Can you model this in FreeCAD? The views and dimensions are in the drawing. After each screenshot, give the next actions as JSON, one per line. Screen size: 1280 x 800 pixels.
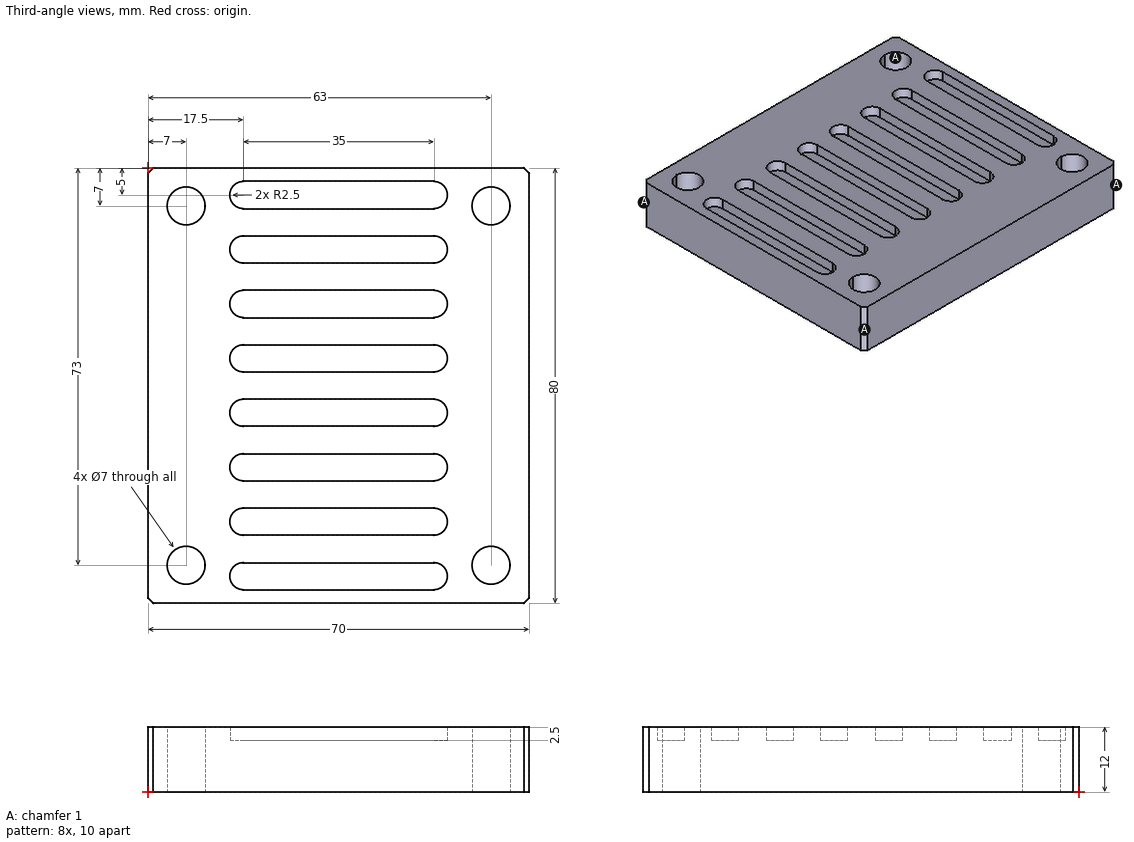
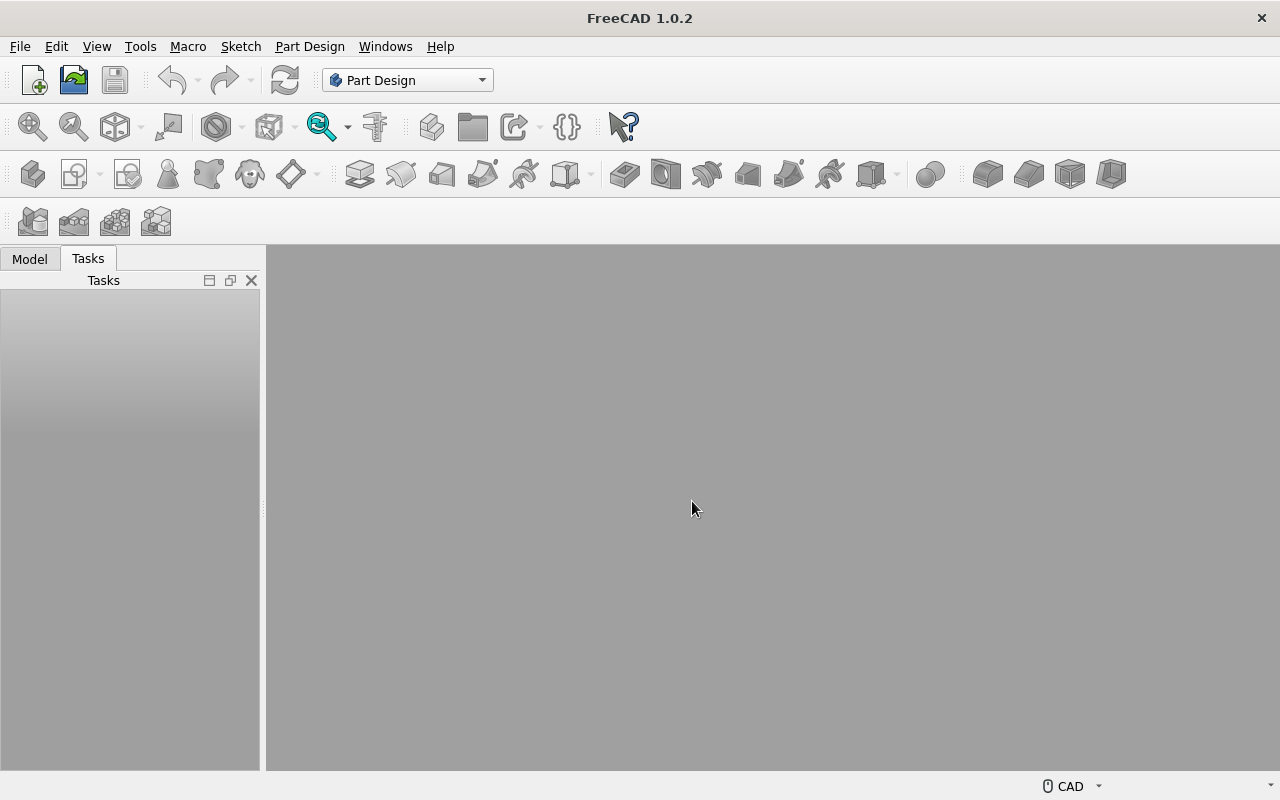
{"action": "key", "text": "ctrl+n"}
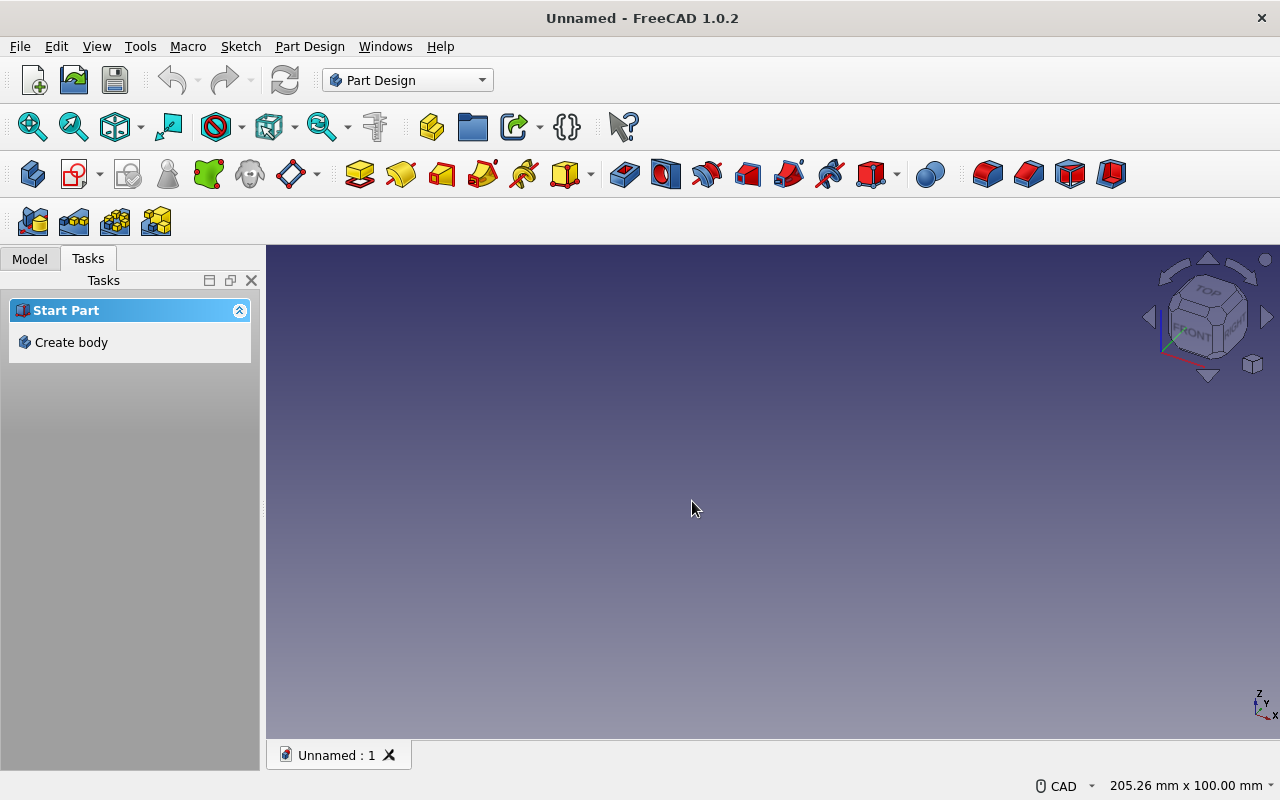
{"action": "left_click", "coordinate": [74, 174]}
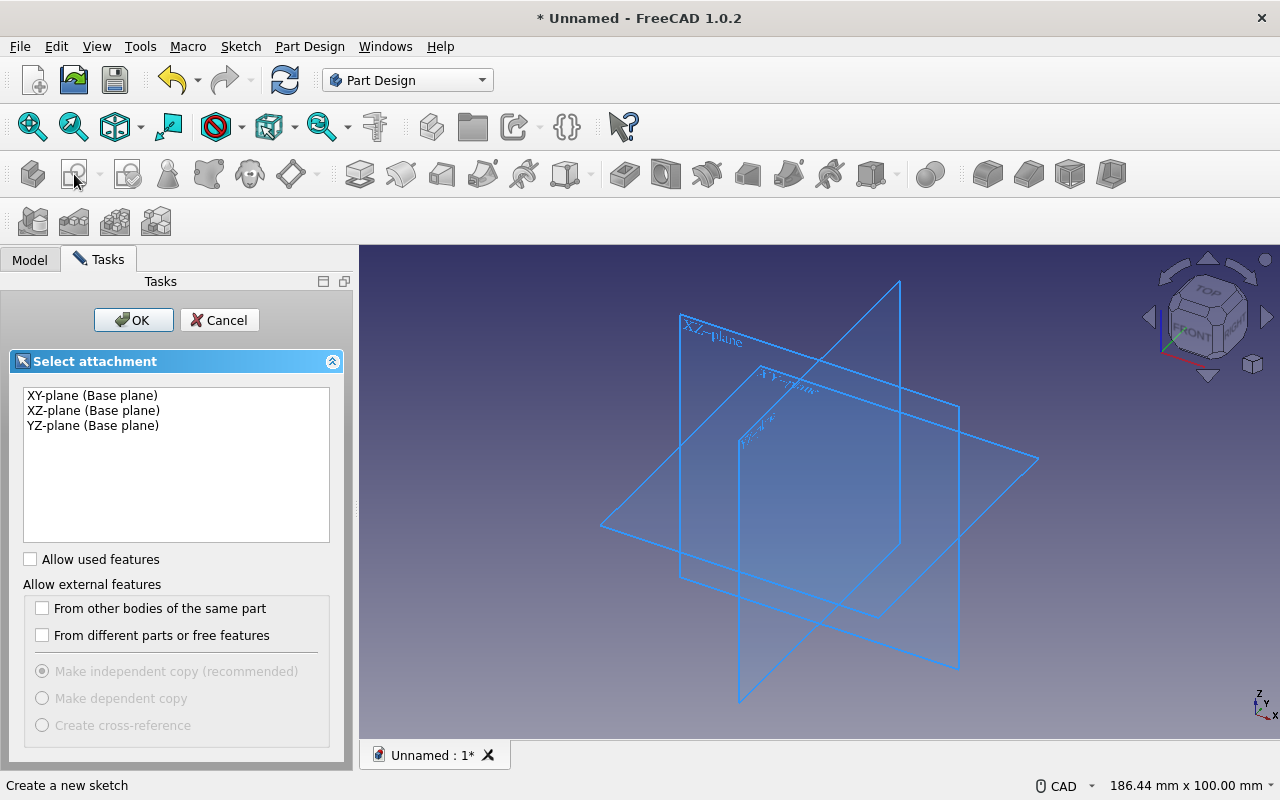
{"action": "left_click", "coordinate": [84, 396]}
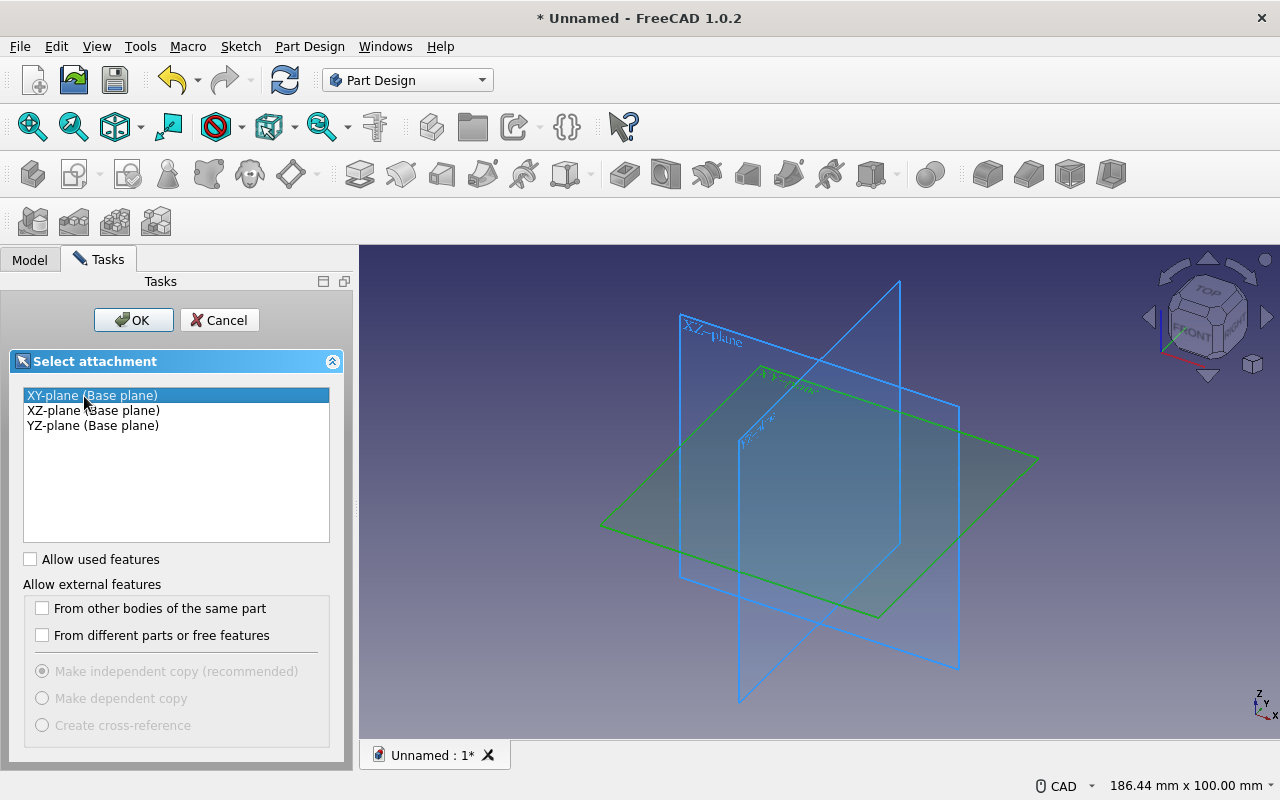
{"action": "left_click", "coordinate": [134, 320]}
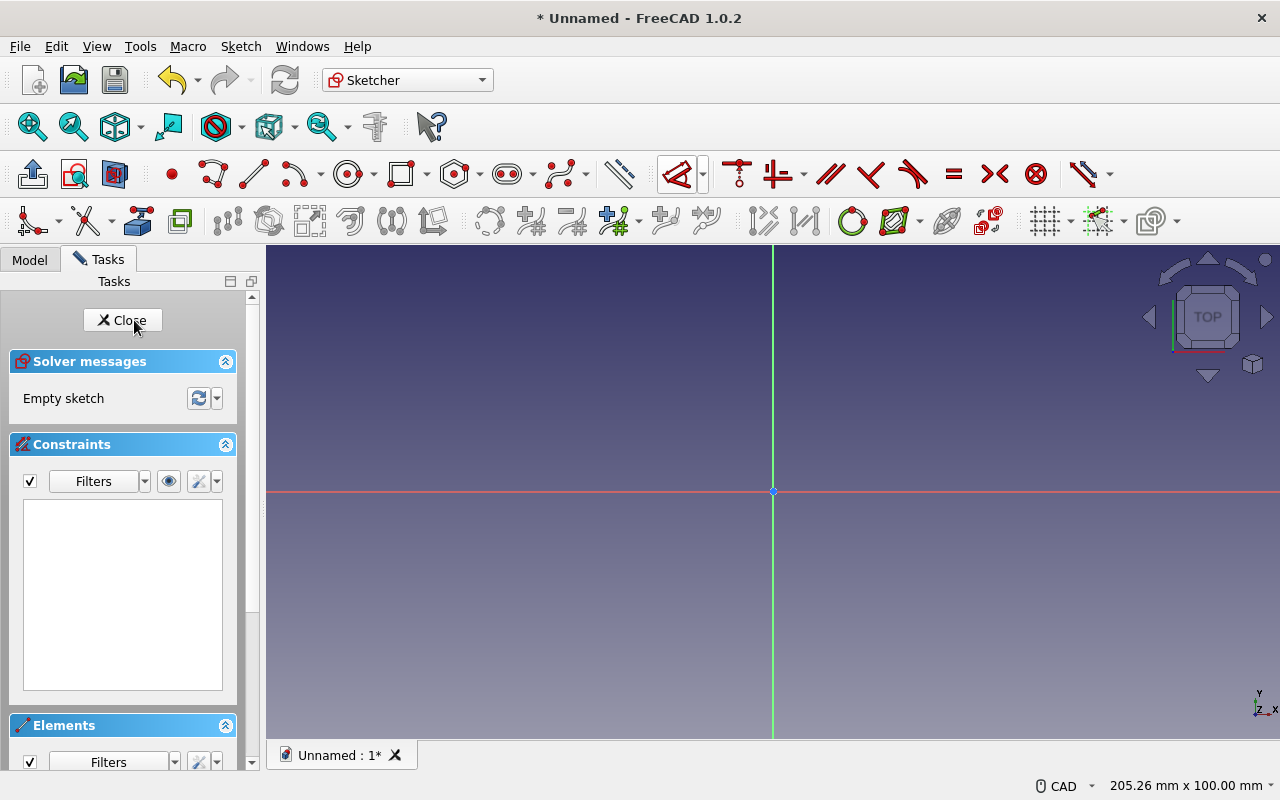
{"action": "scroll", "coordinate": [294, 273], "scroll_direction": "down", "scroll_amount": 2}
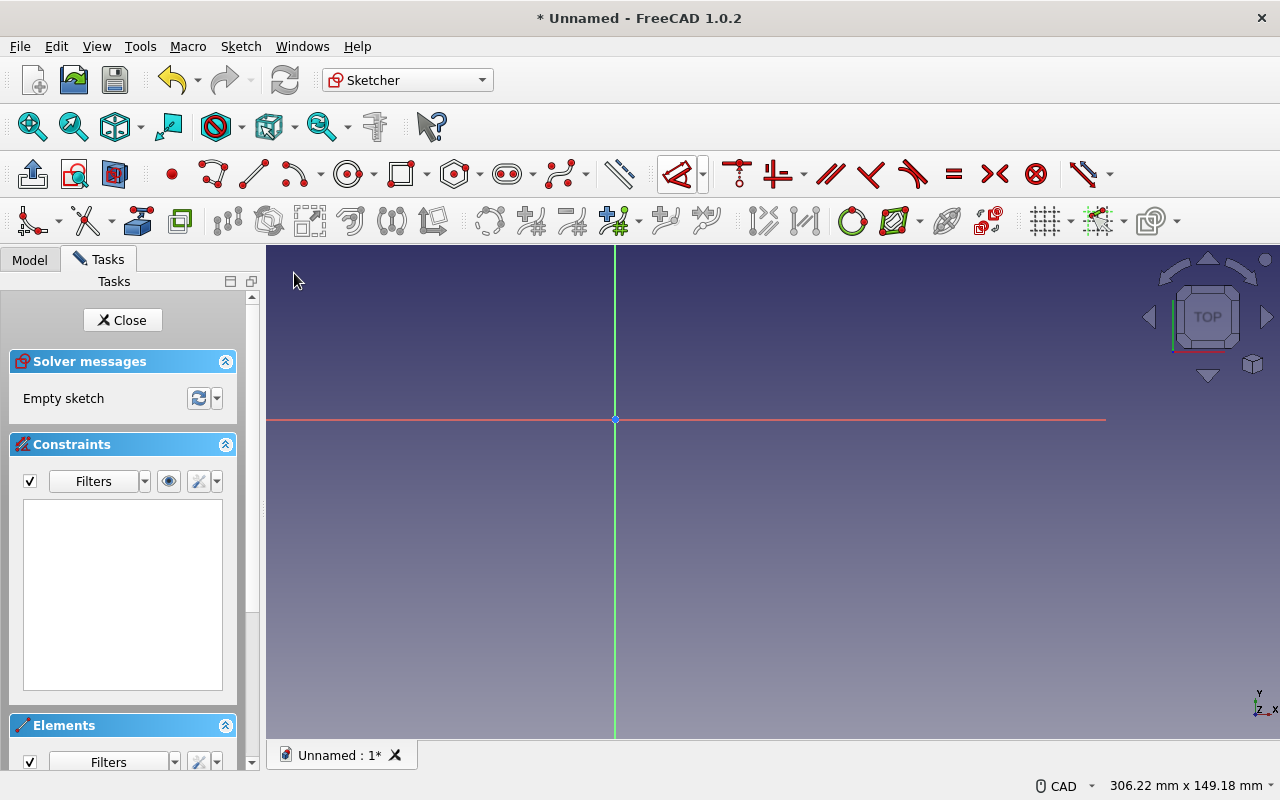
{"action": "key", "text": "g r"}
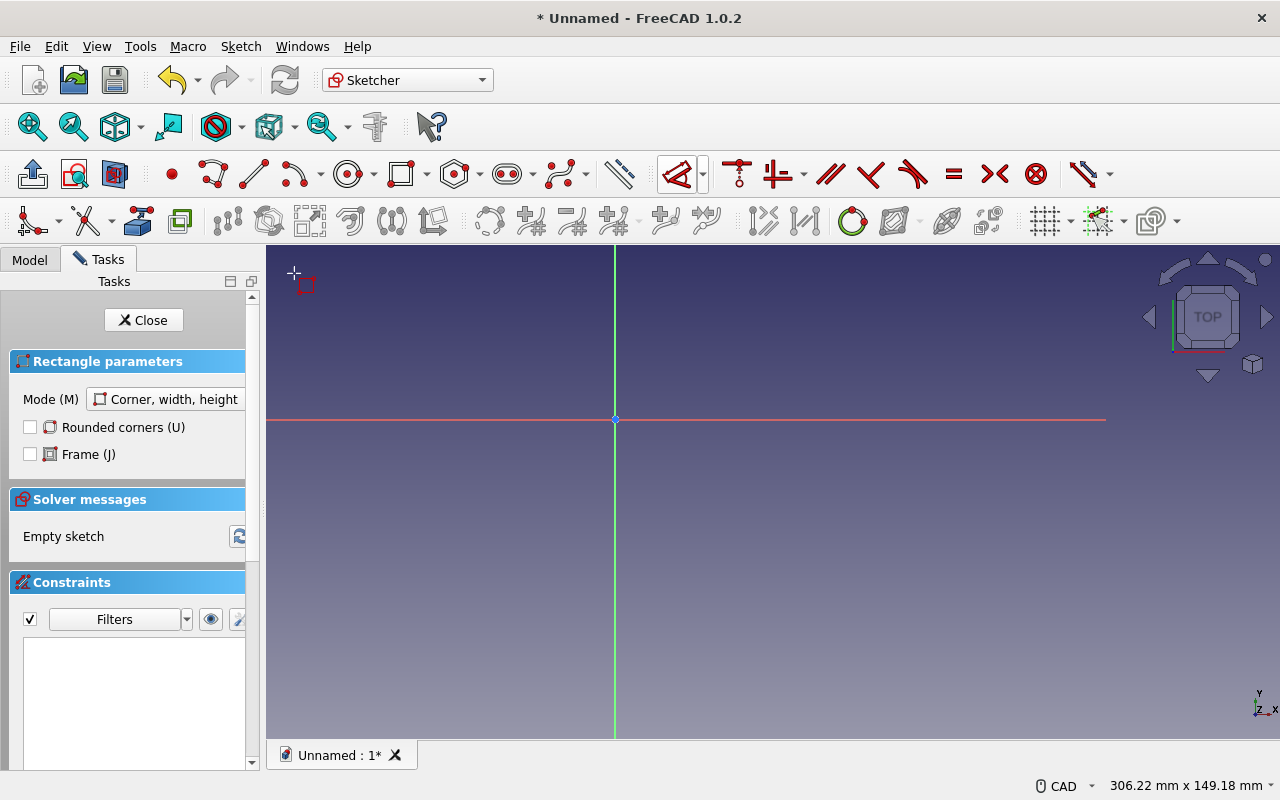
{"action": "left_click", "coordinate": [615, 420]}
{"action": "mouse_move", "coordinate": [847, 685]}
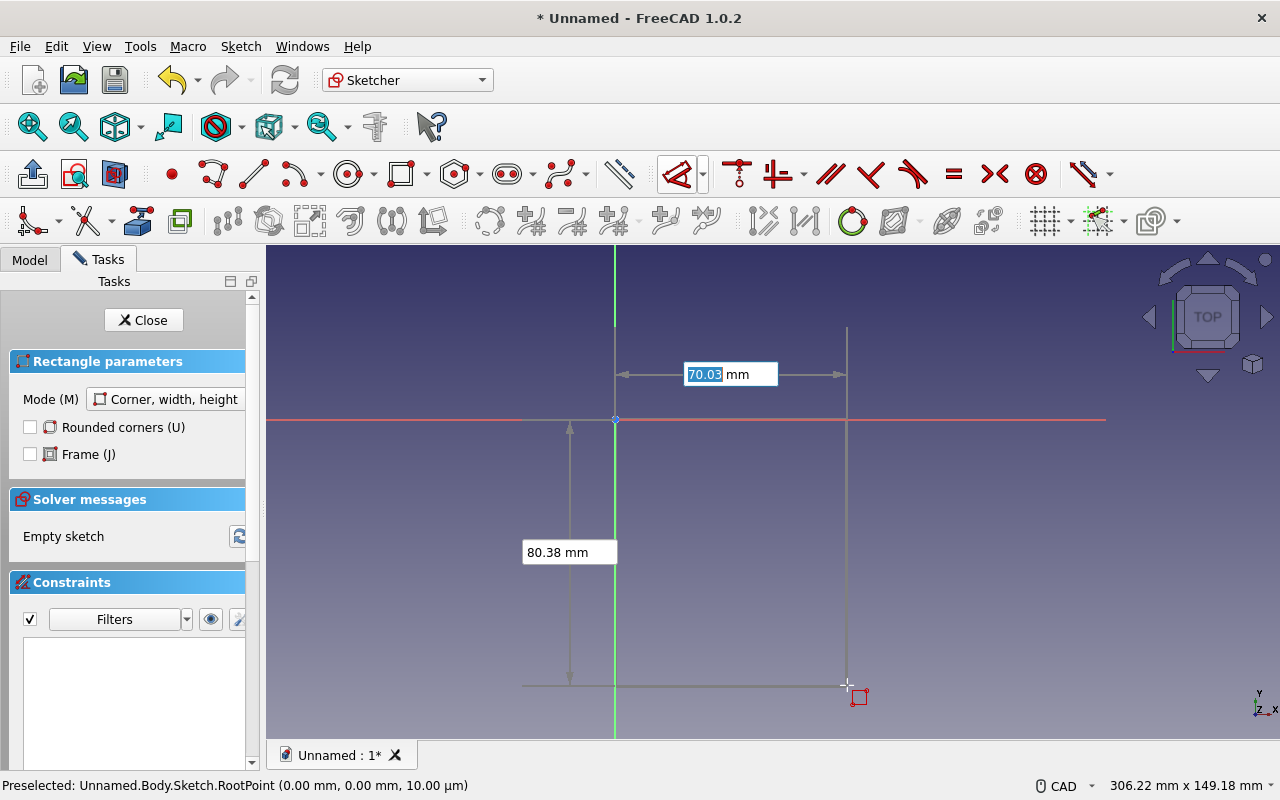
{"action": "type", "text": "70"}
{"action": "key", "text": "Tab"}
{"action": "type", "text": "80"}
{"action": "key", "text": "Return"}
{"action": "key", "text": "Escape"}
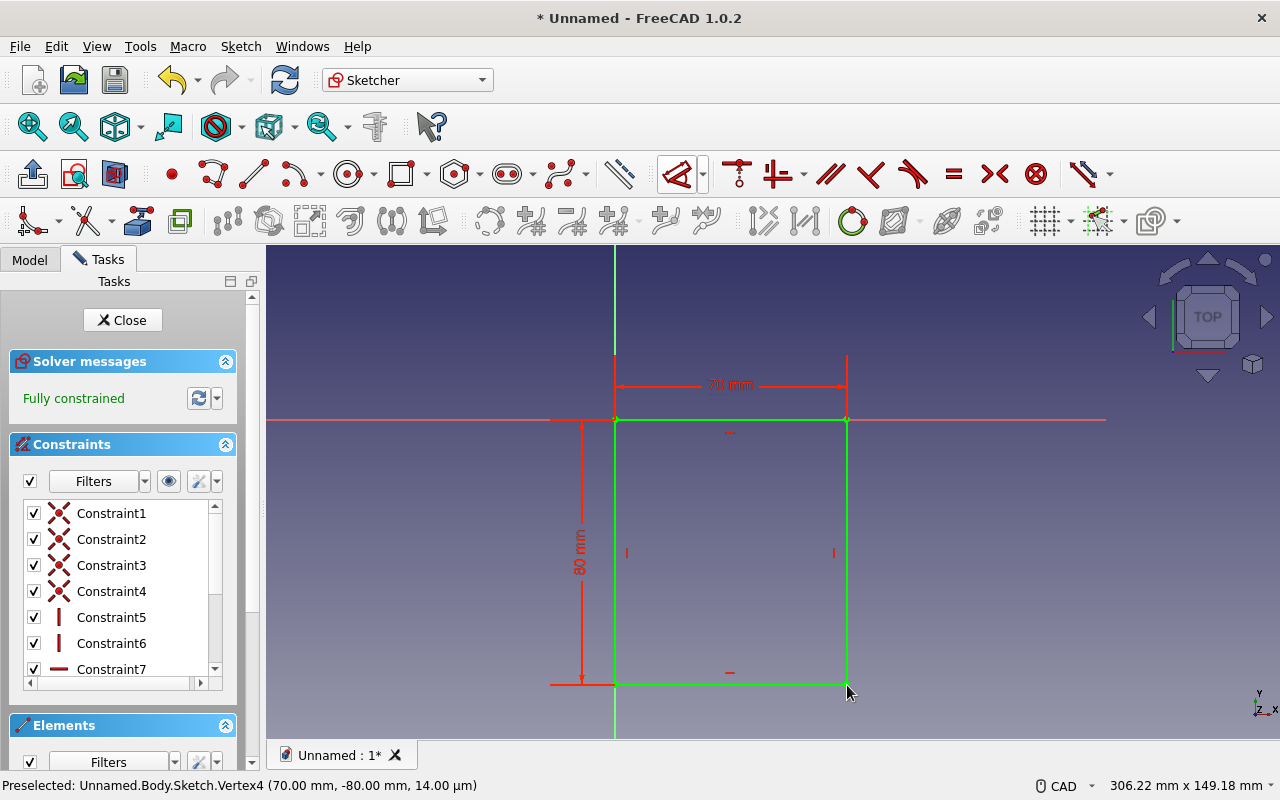
{"action": "left_click", "coordinate": [123, 320]}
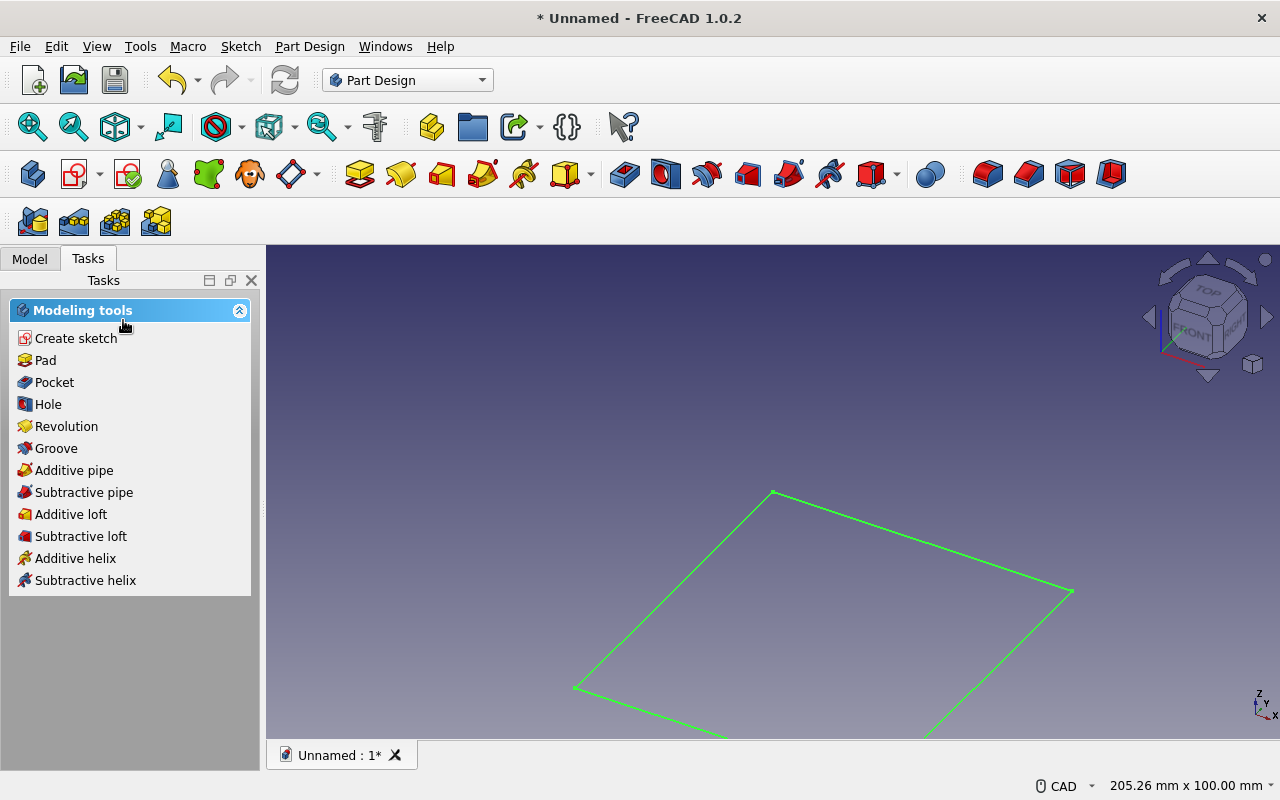
{"action": "left_click", "coordinate": [360, 174]}